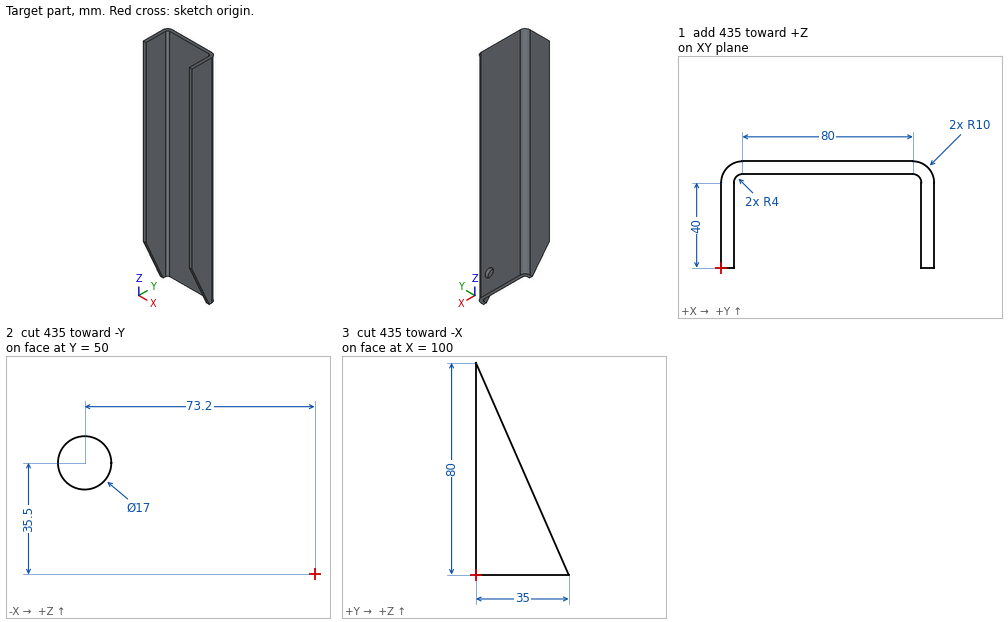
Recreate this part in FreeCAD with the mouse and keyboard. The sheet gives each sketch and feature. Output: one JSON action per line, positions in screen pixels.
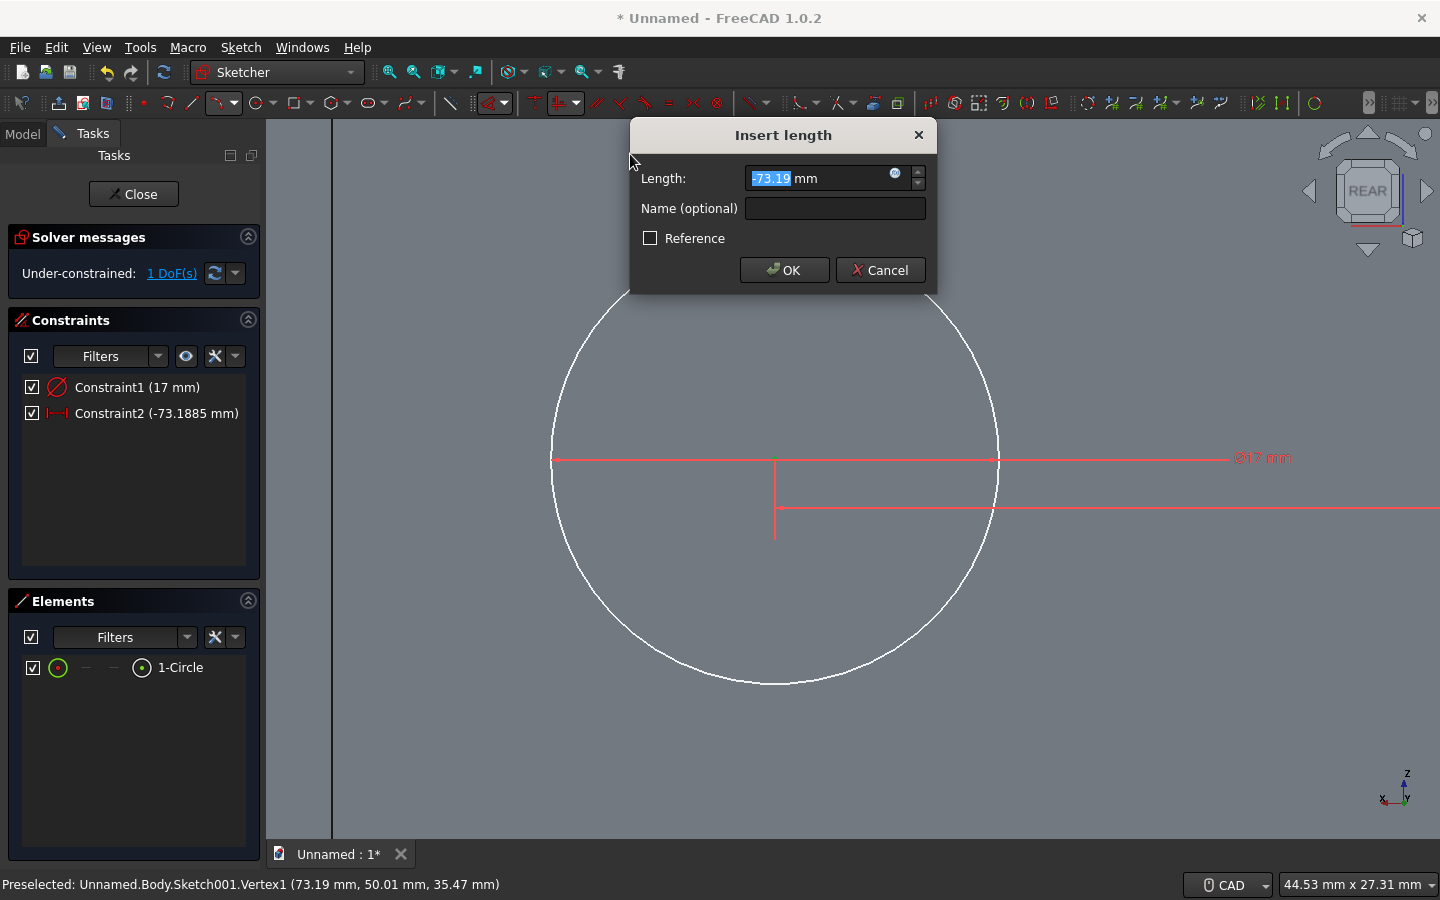
{"action": "type", "text": "-73.2"}
{"action": "key", "text": "Return"}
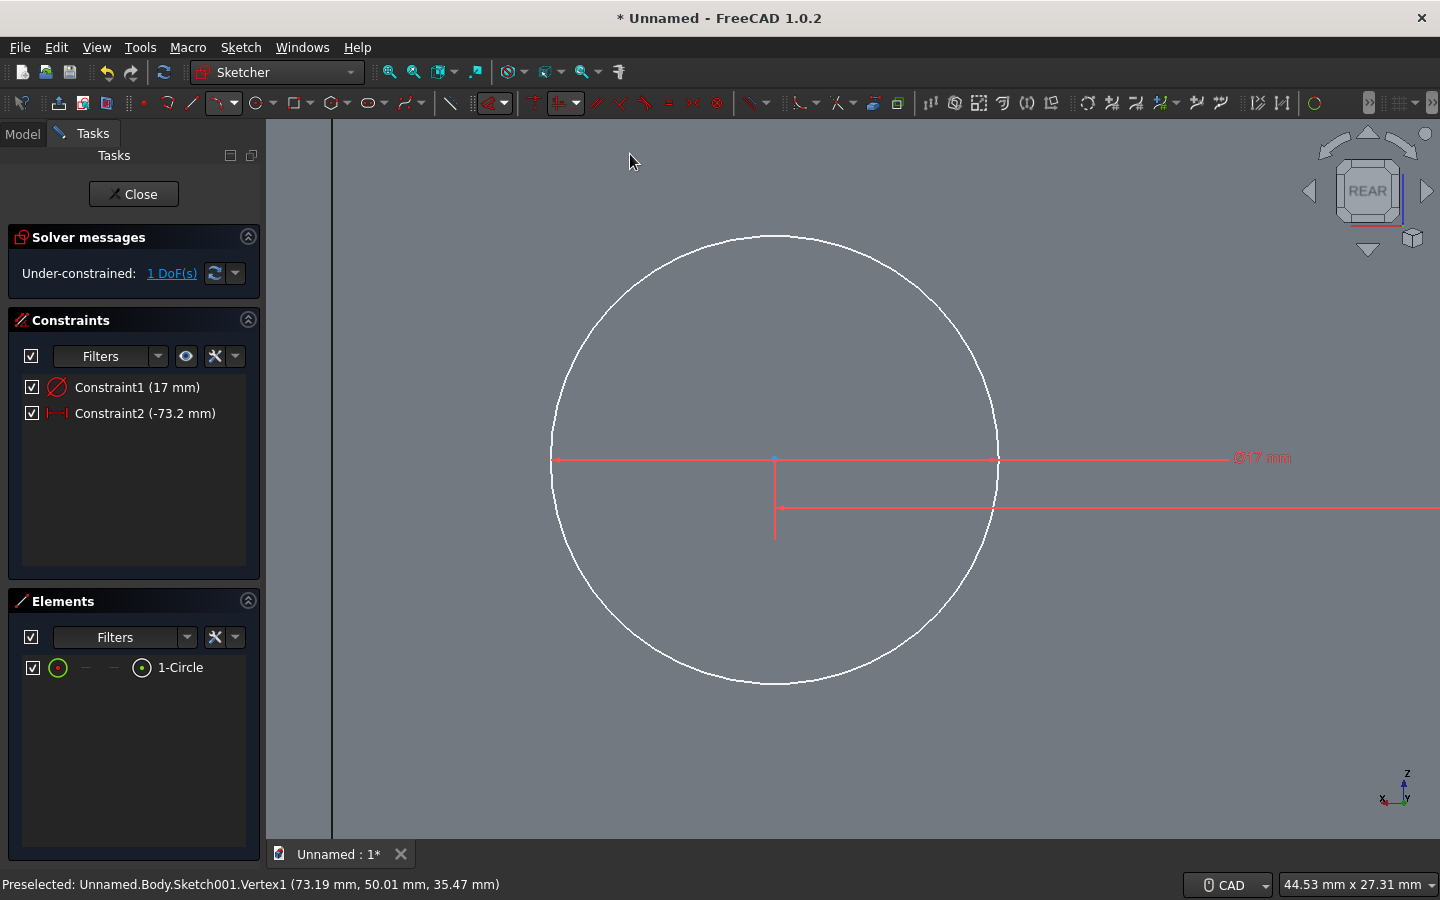
{"action": "left_click", "coordinate": [775, 460]}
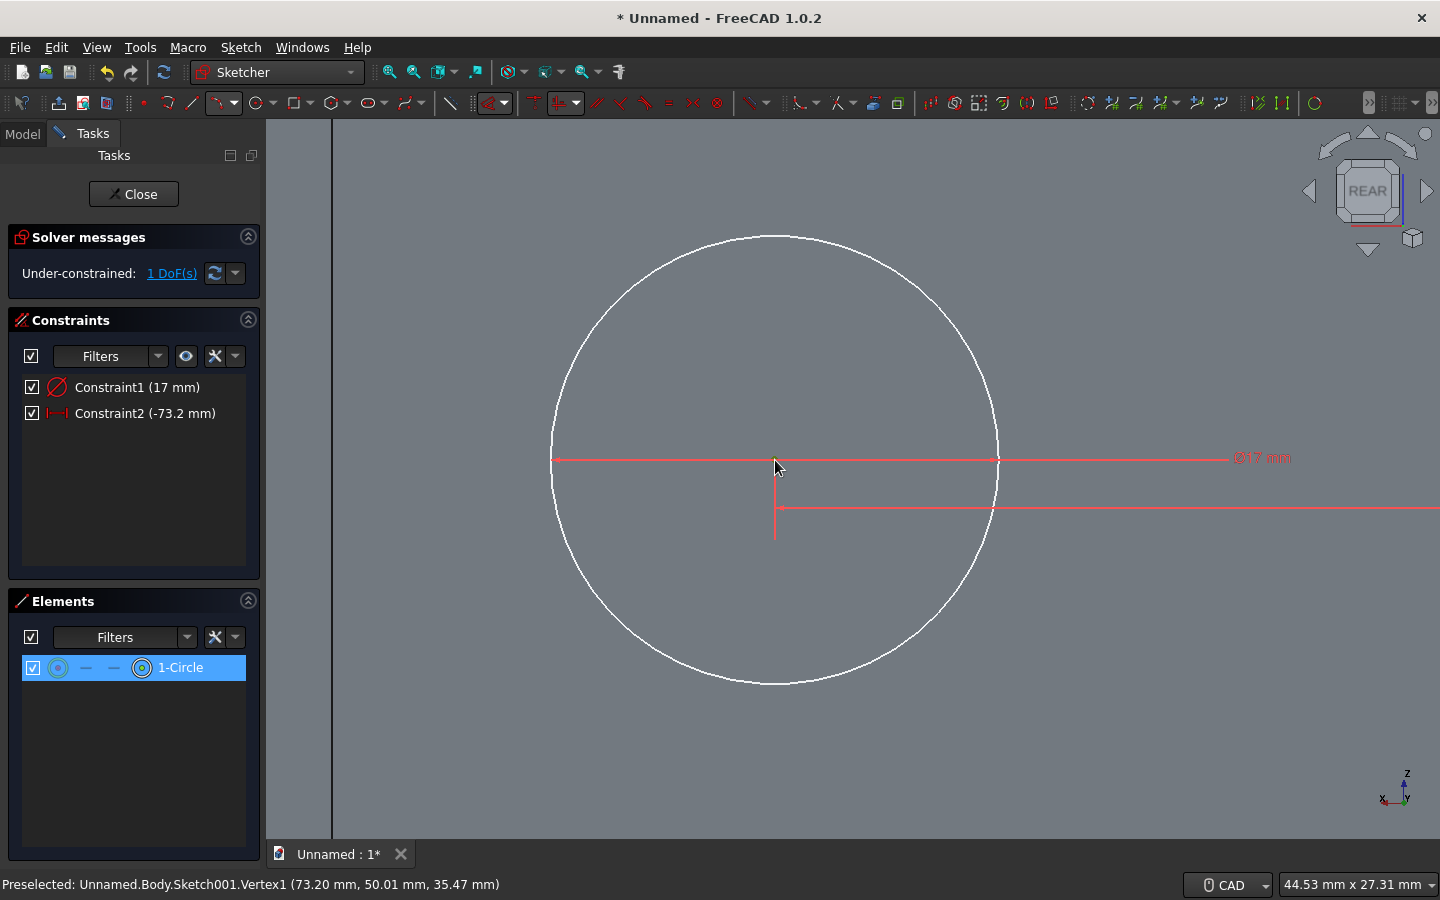
{"action": "key", "text": "i"}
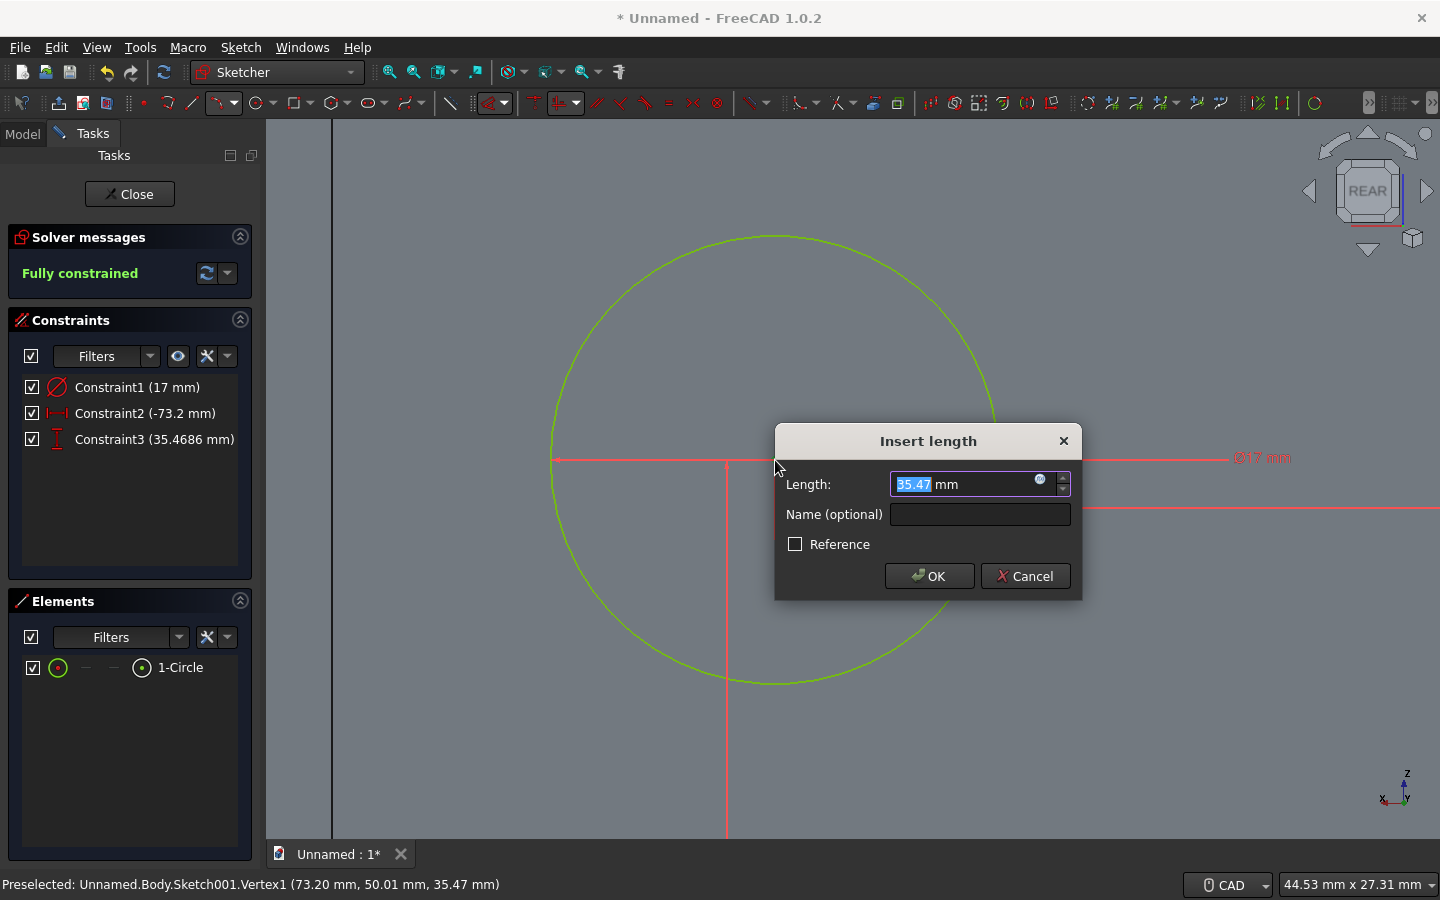
{"action": "type", "text": "35.5"}
{"action": "key", "text": "Return"}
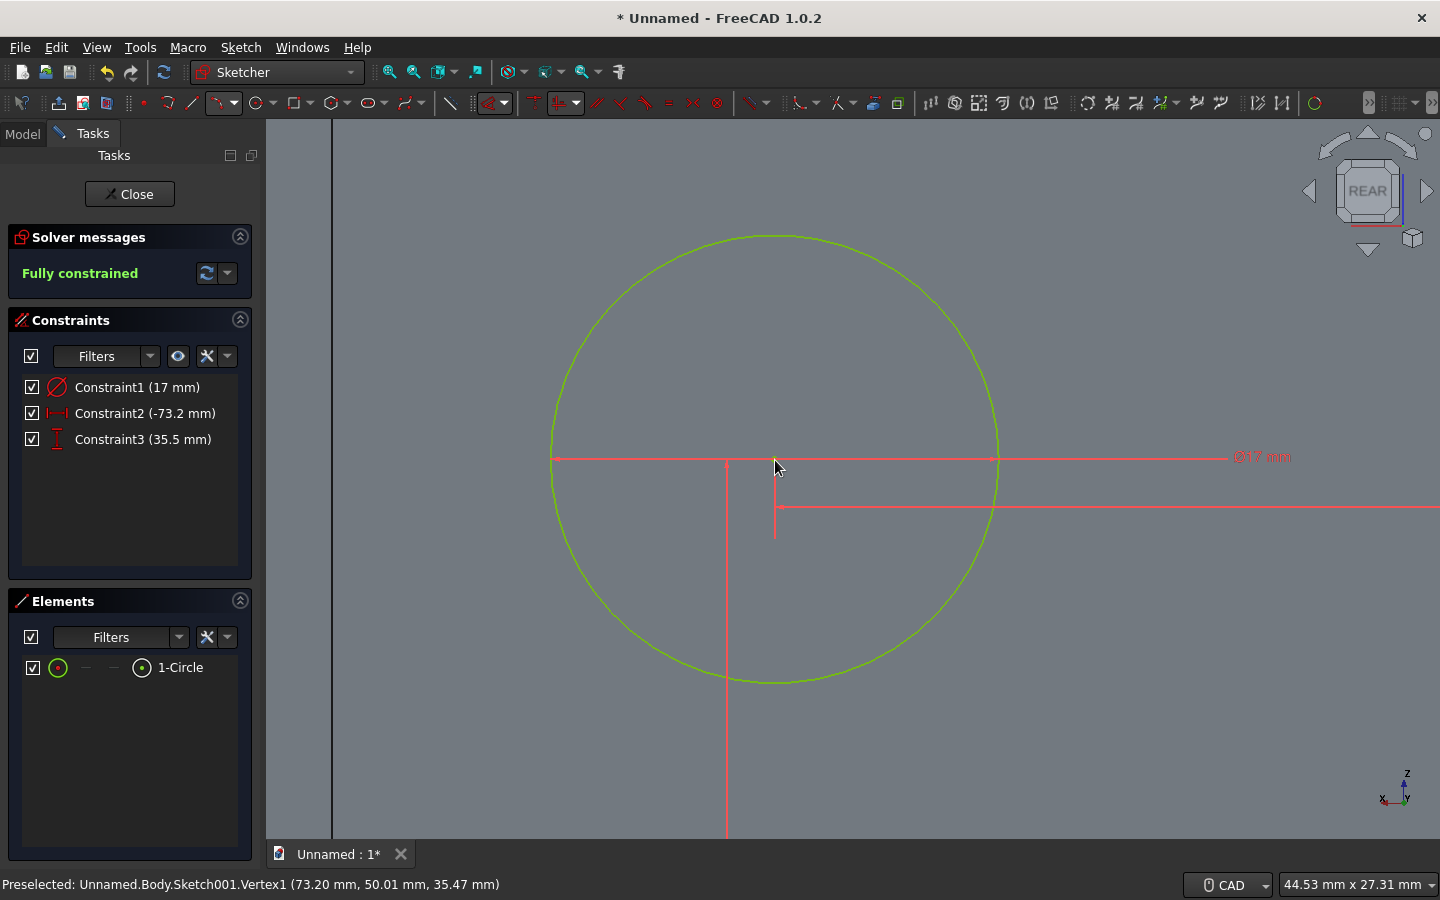
{"action": "left_click", "coordinate": [130, 194]}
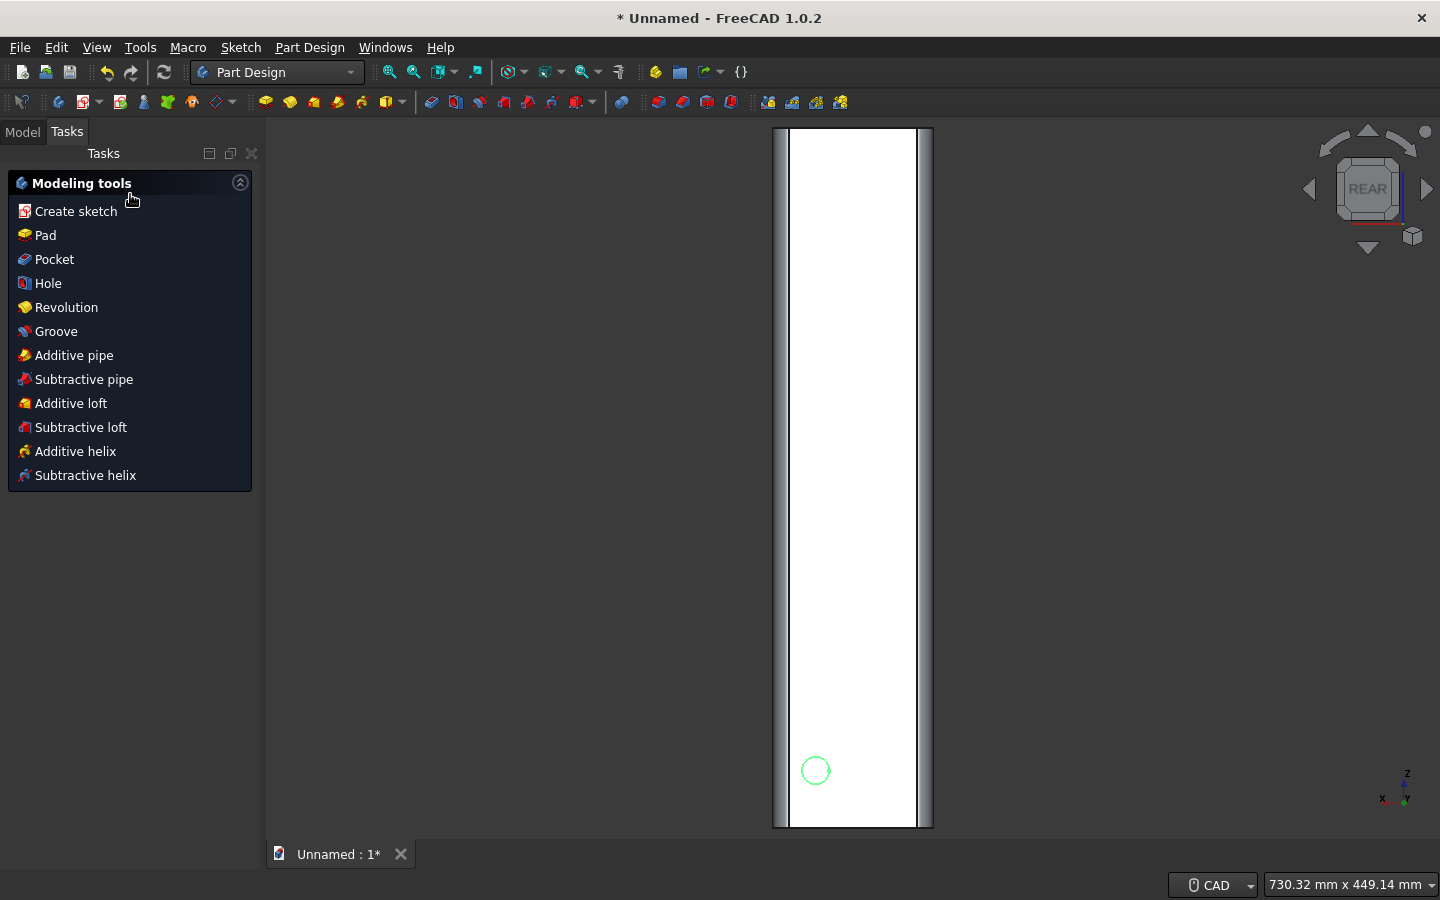
{"action": "left_click", "coordinate": [432, 102]}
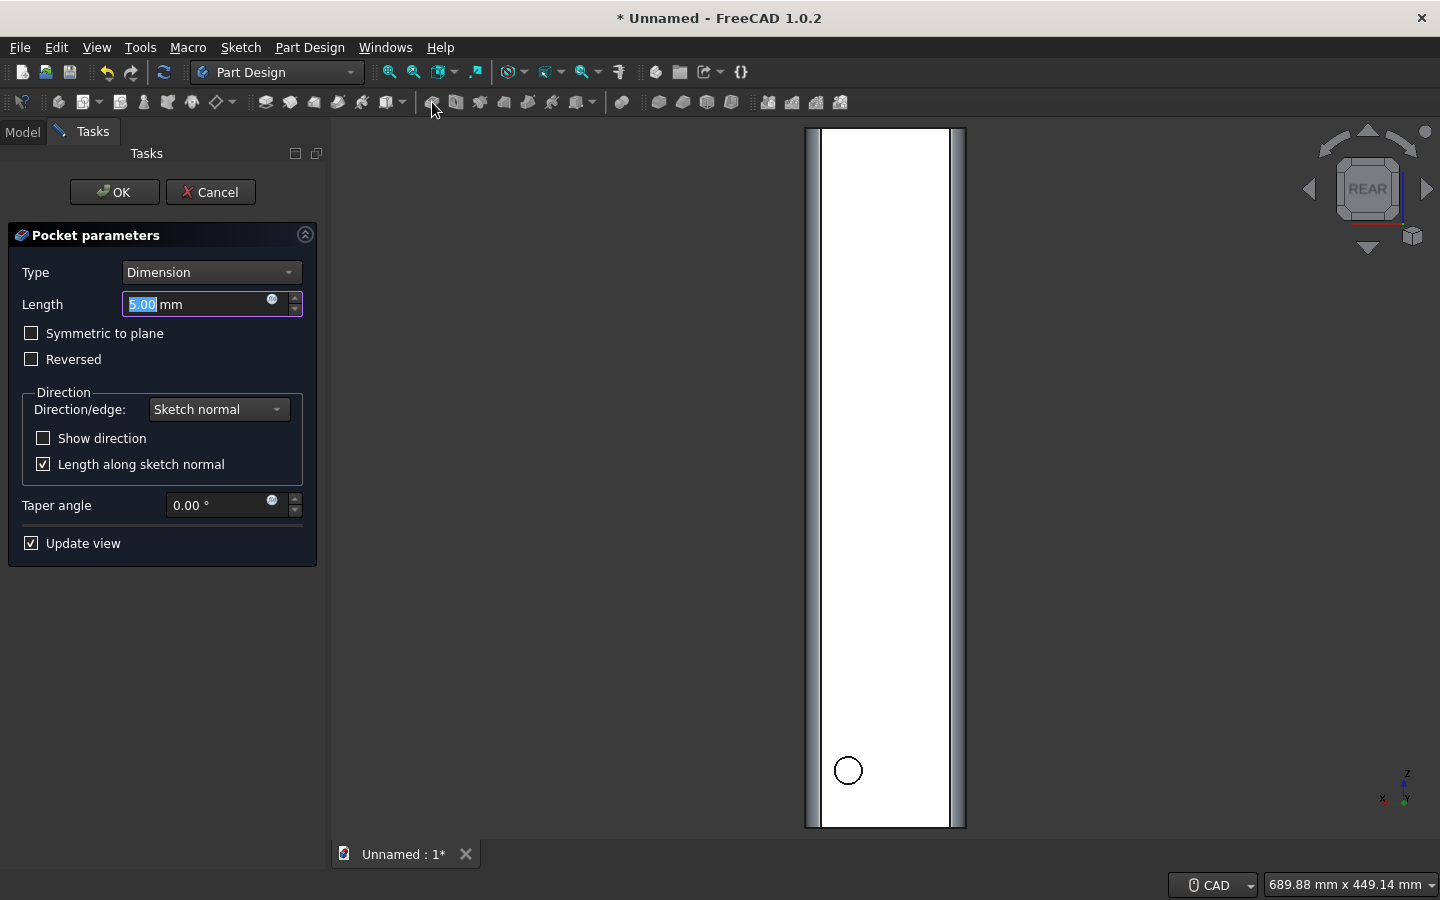
{"action": "type", "text": "435"}
{"action": "key", "text": "Tab"}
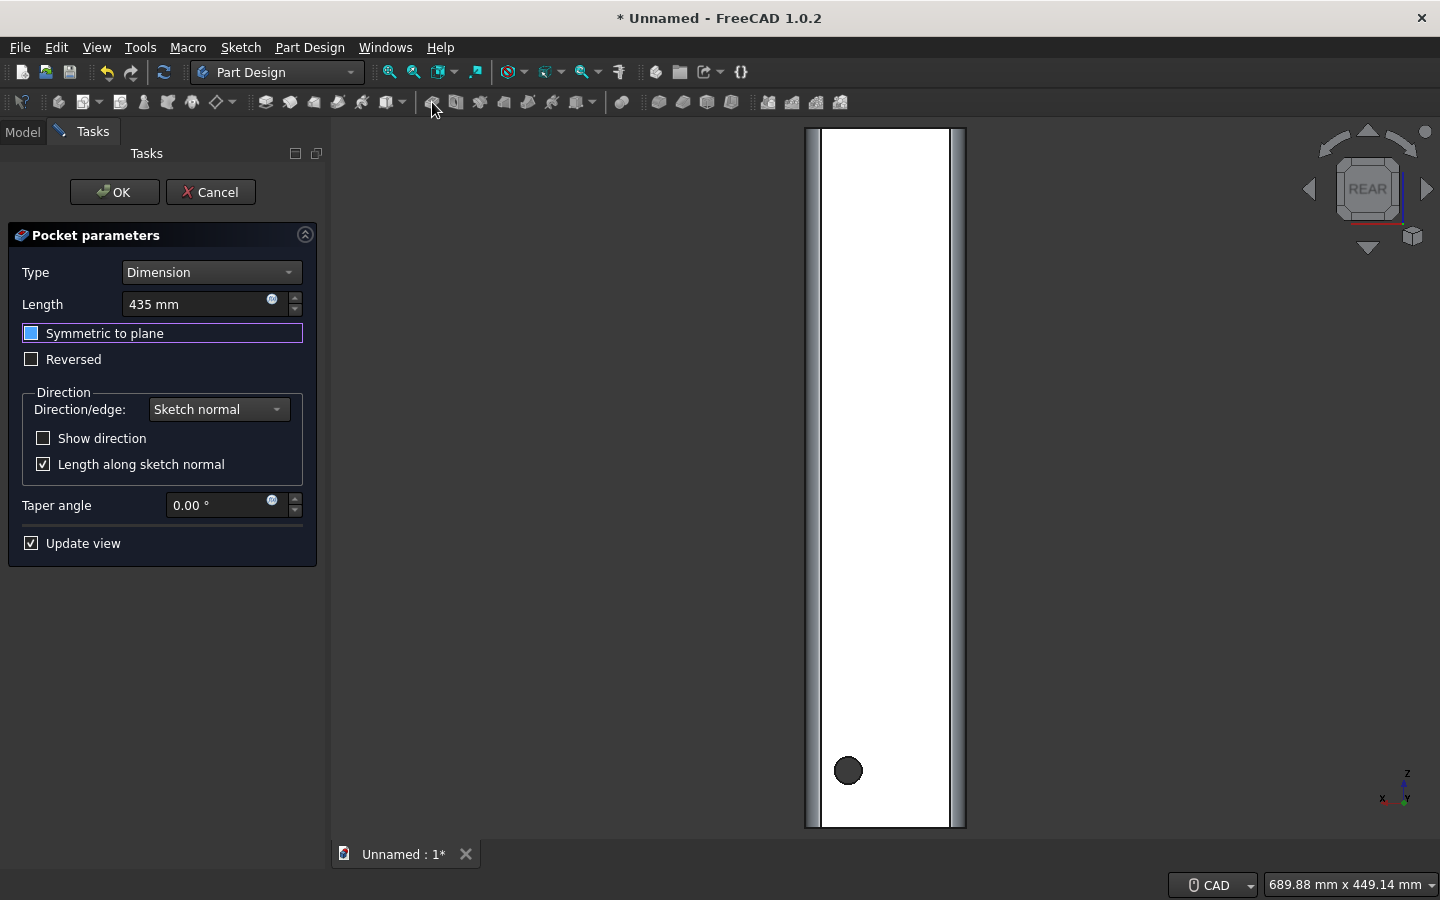
{"action": "left_click", "coordinate": [115, 192]}